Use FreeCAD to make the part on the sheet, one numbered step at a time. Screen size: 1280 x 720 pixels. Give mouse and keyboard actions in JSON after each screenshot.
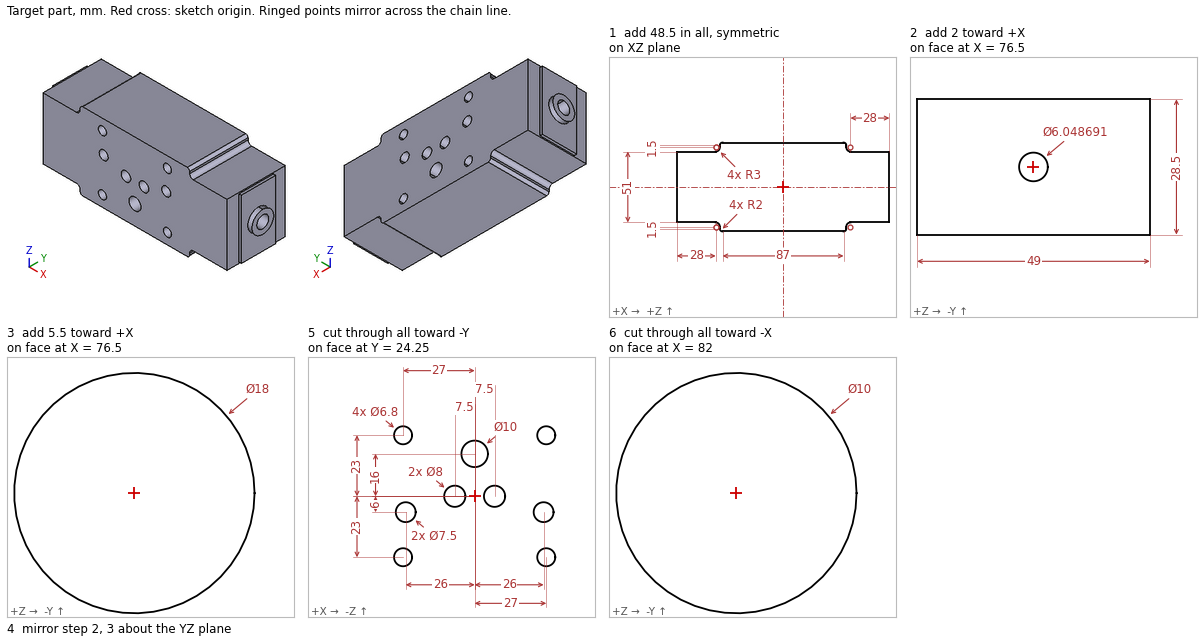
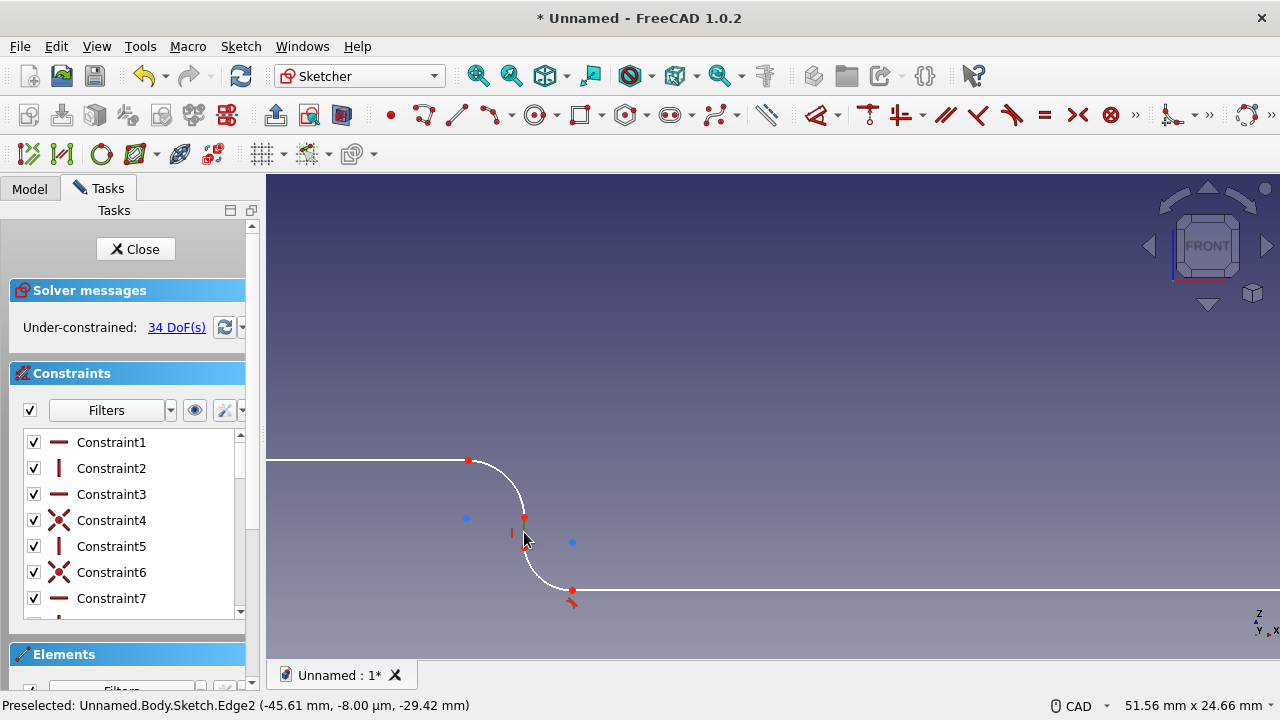
{"action": "left_click", "coordinate": [531, 567]}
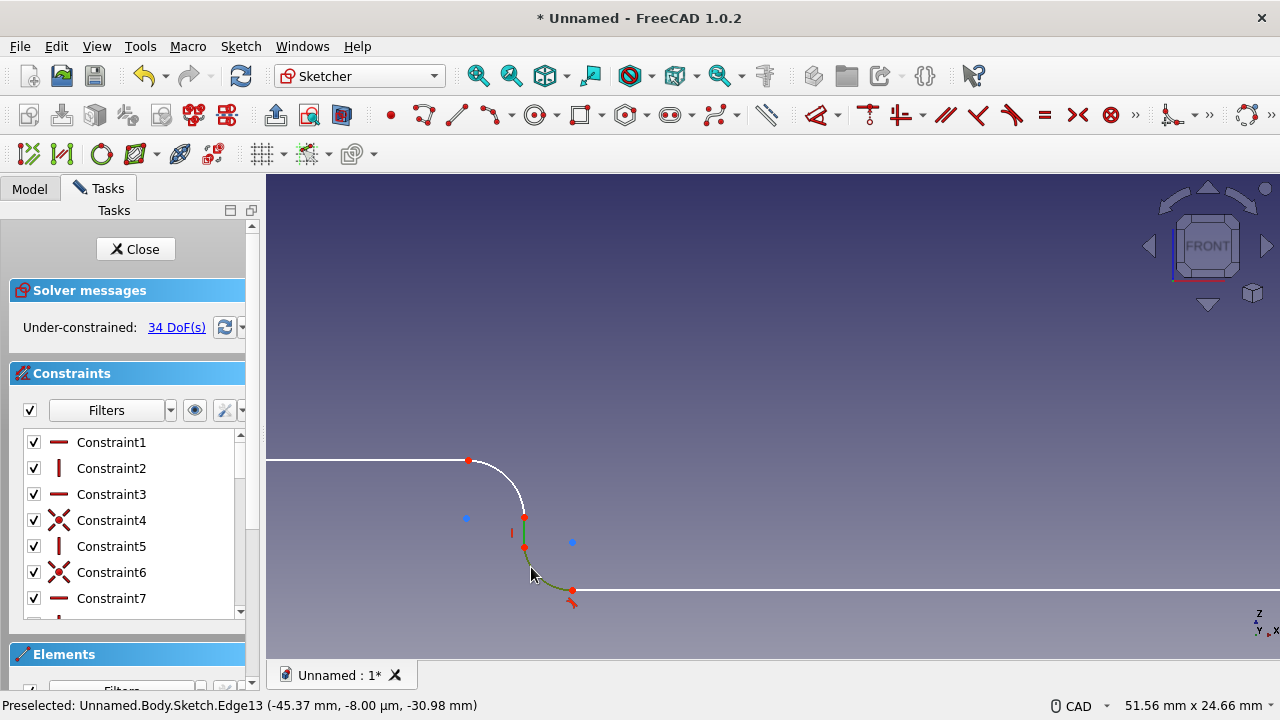
{"action": "left_click", "coordinate": [1012, 116]}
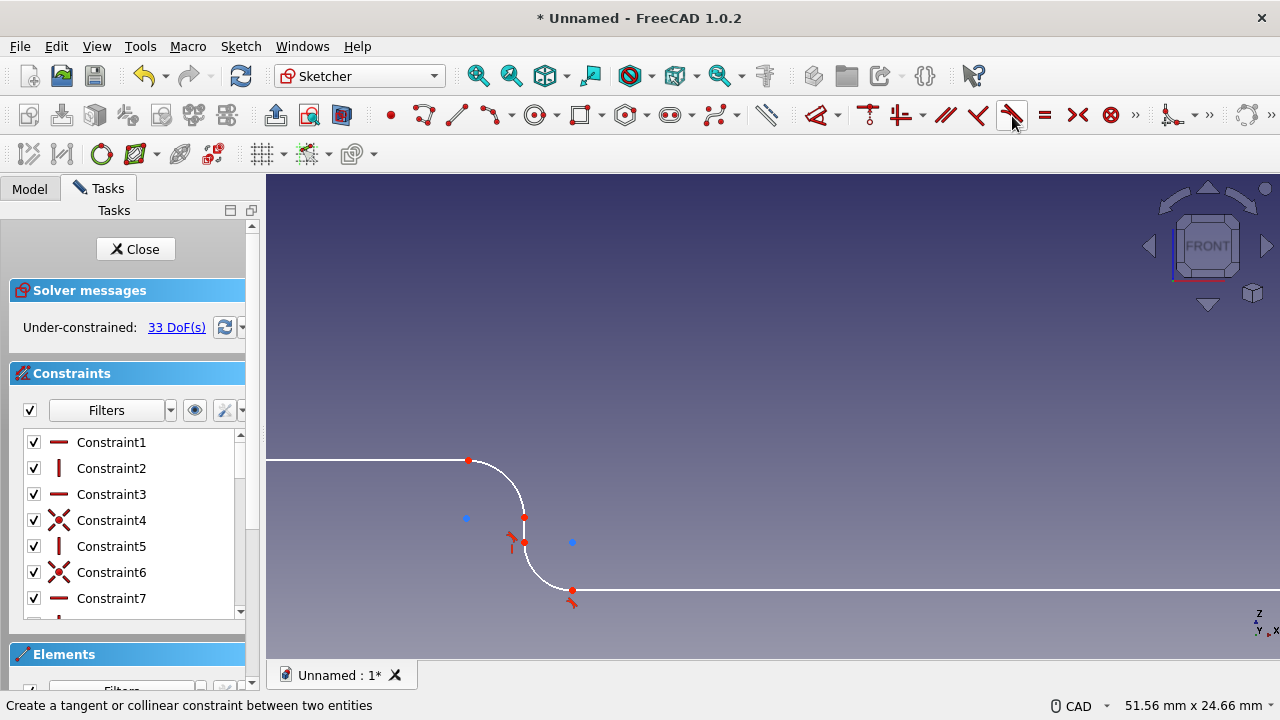
{"action": "scroll", "coordinate": [524, 532], "scroll_direction": "up", "scroll_amount": 2}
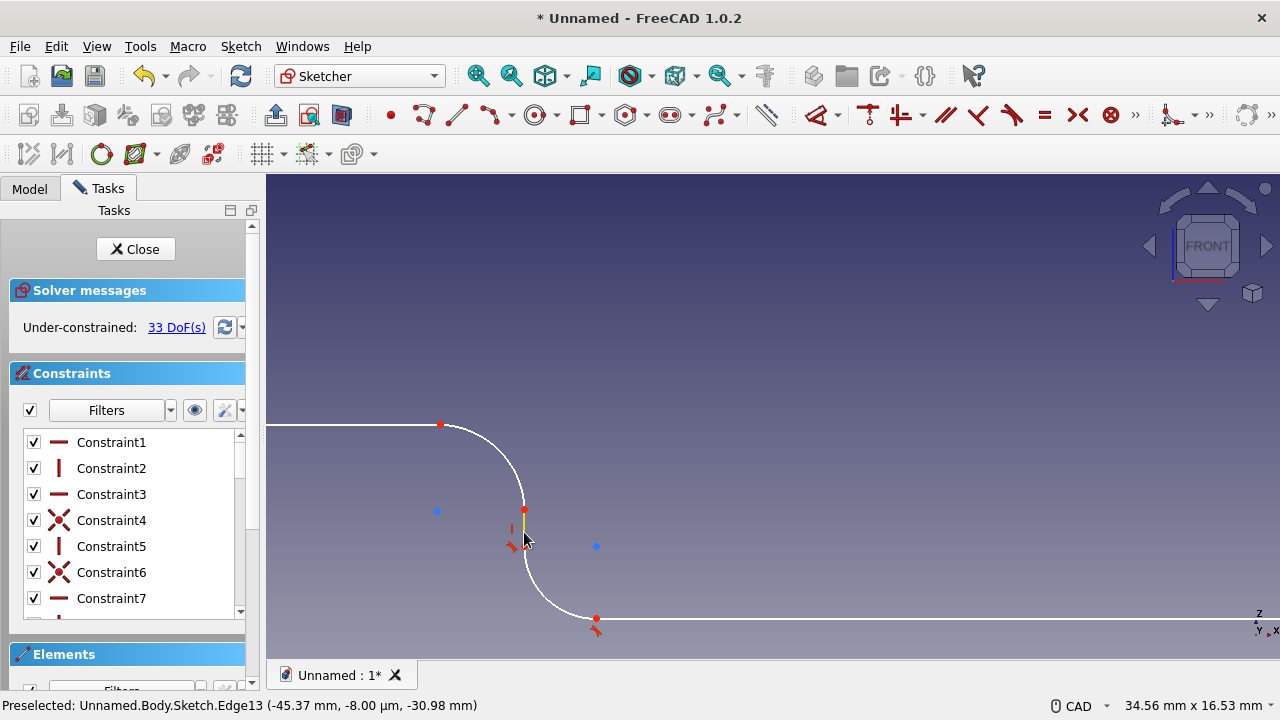
{"action": "left_click", "coordinate": [524, 532]}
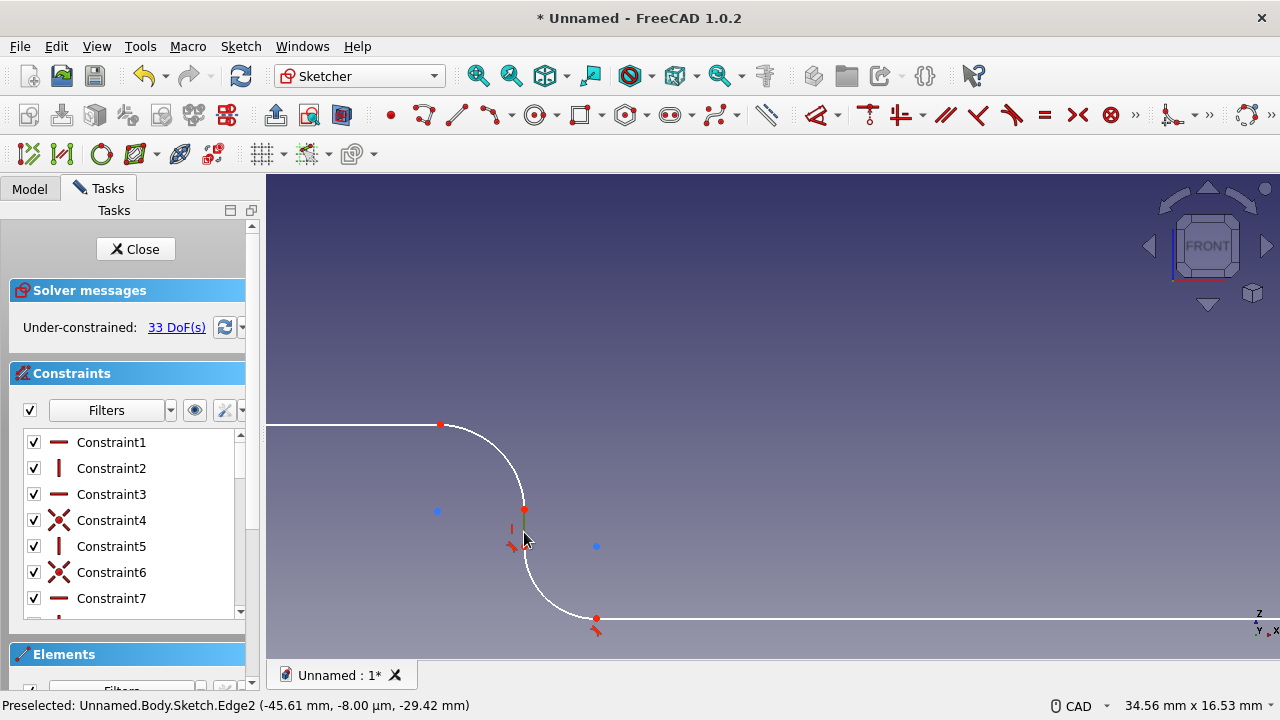
{"action": "left_click", "coordinate": [515, 472]}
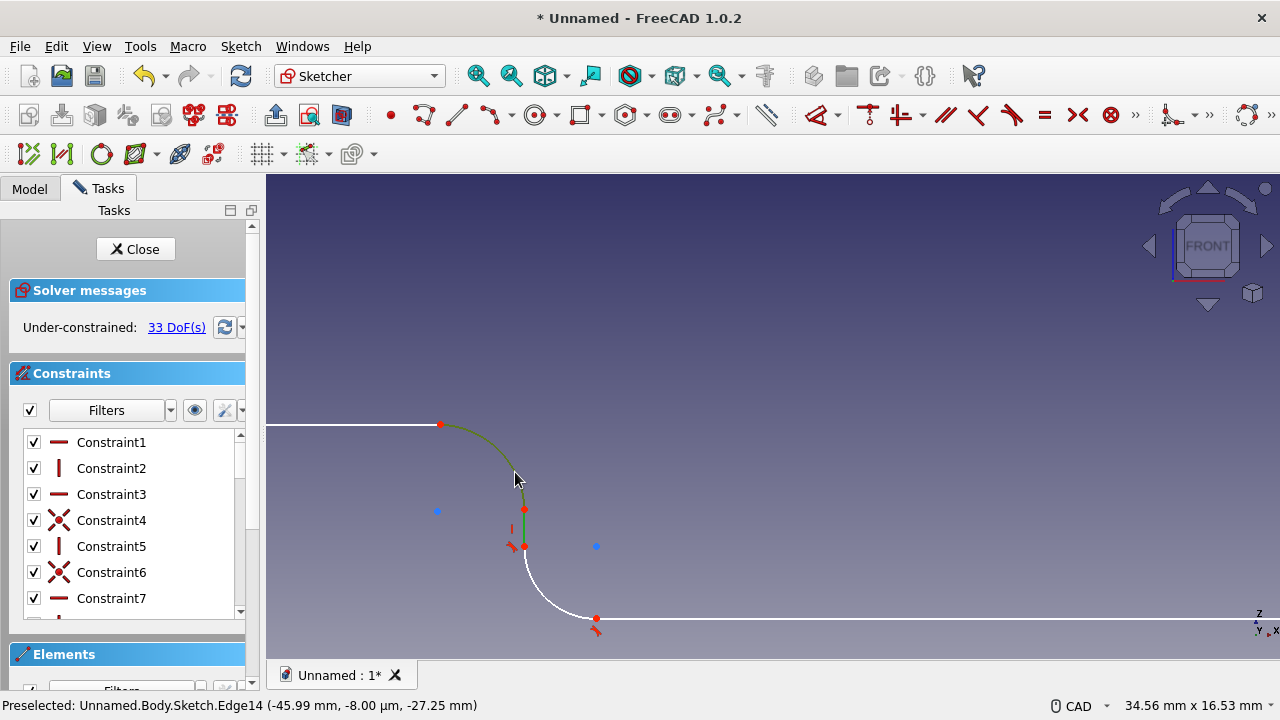
{"action": "left_click", "coordinate": [1012, 116]}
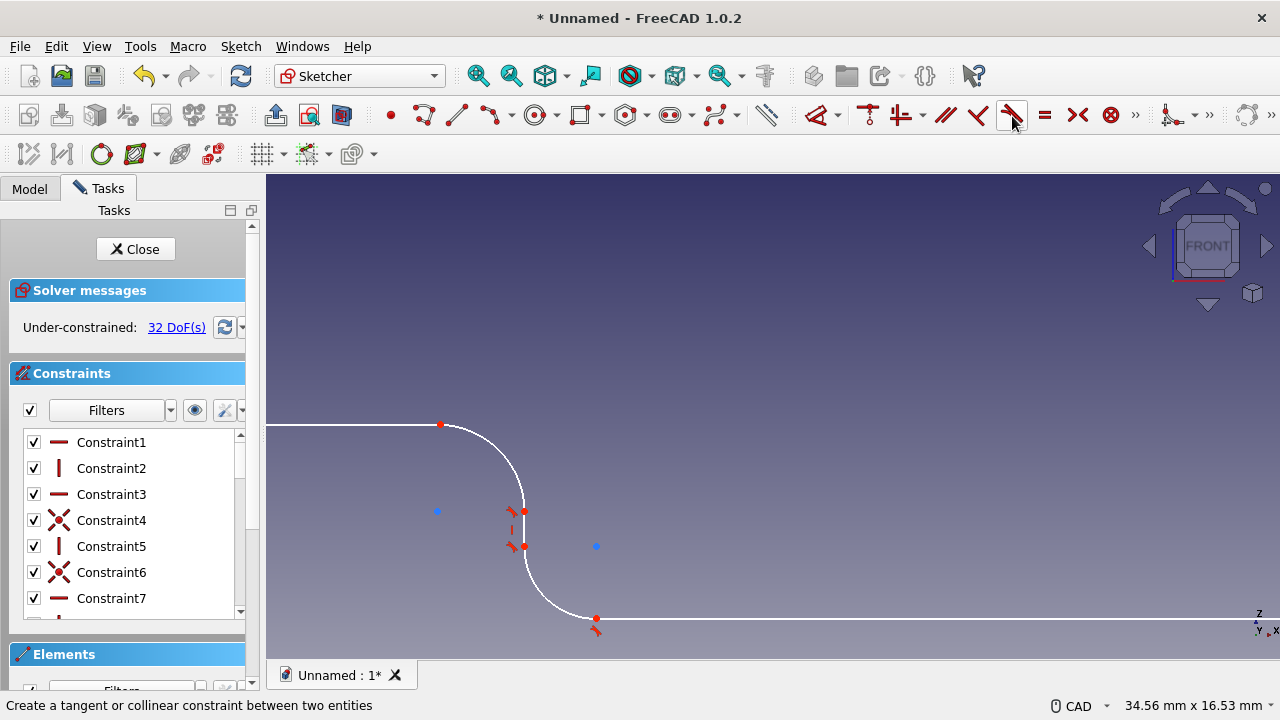
{"action": "scroll", "coordinate": [523, 533], "scroll_direction": "down", "scroll_amount": 10}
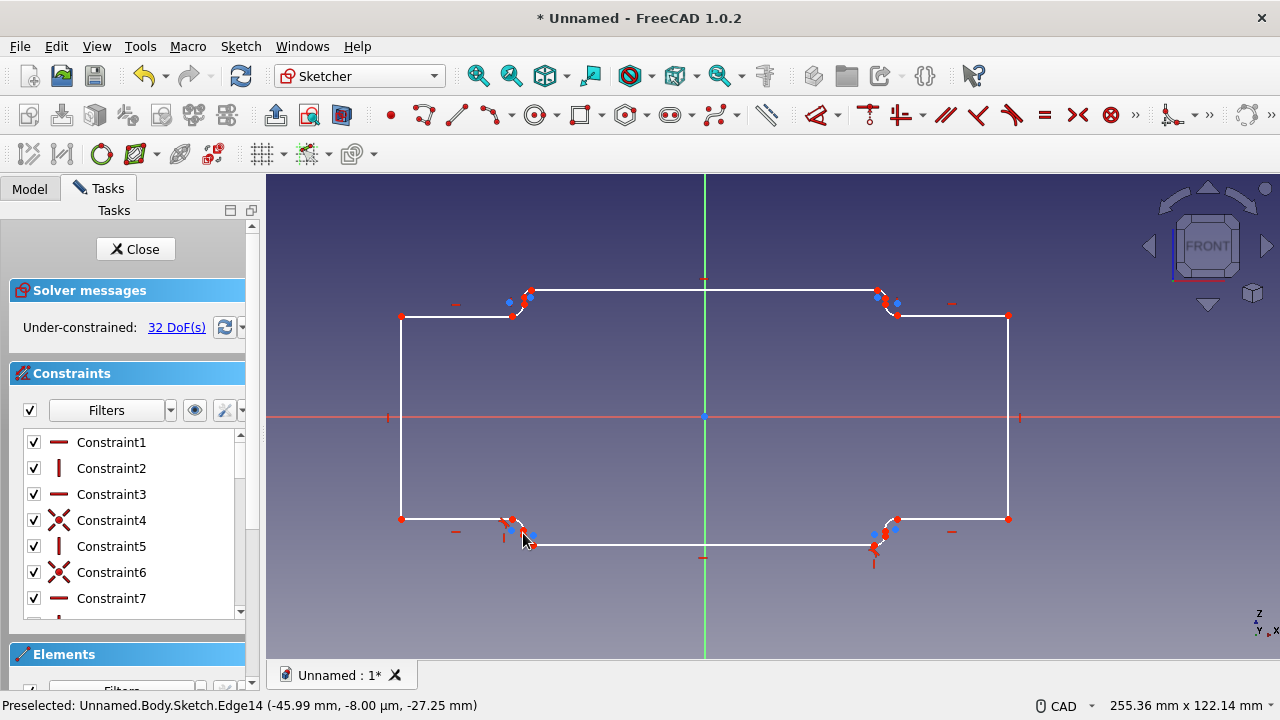
{"action": "left_click", "coordinate": [479, 519]}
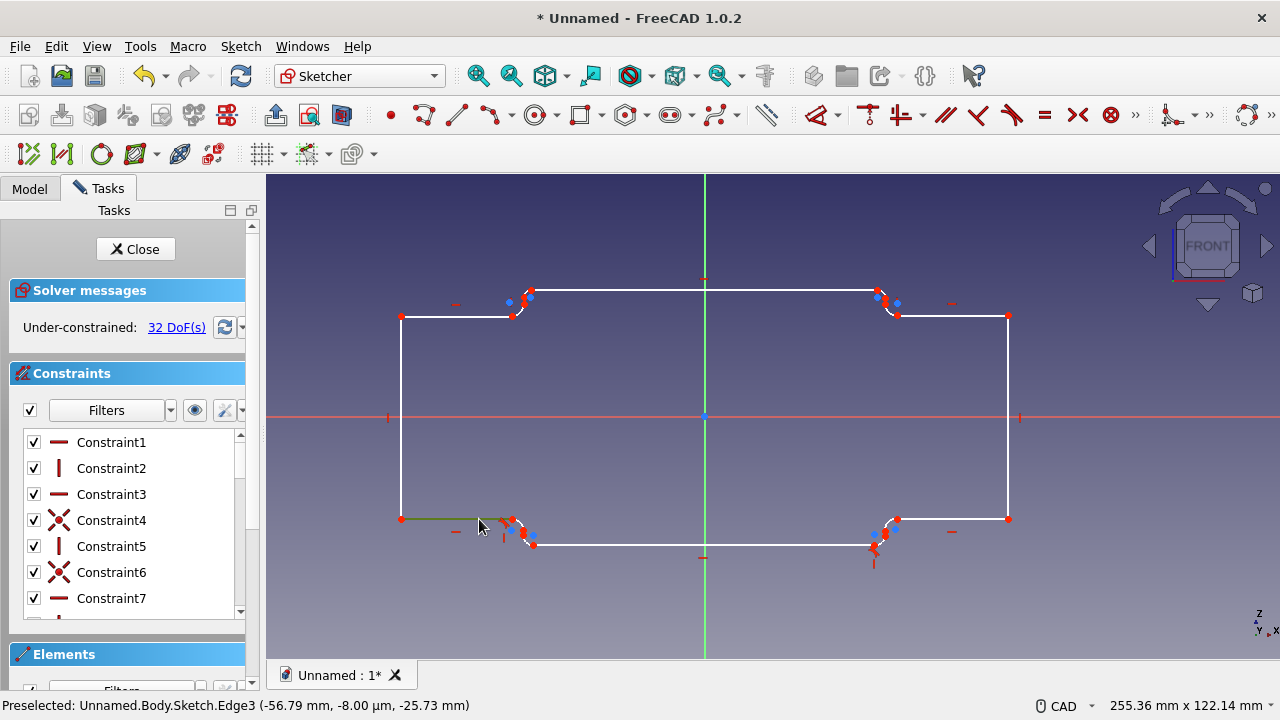
{"action": "scroll", "coordinate": [520, 523], "scroll_direction": "up", "scroll_amount": 3}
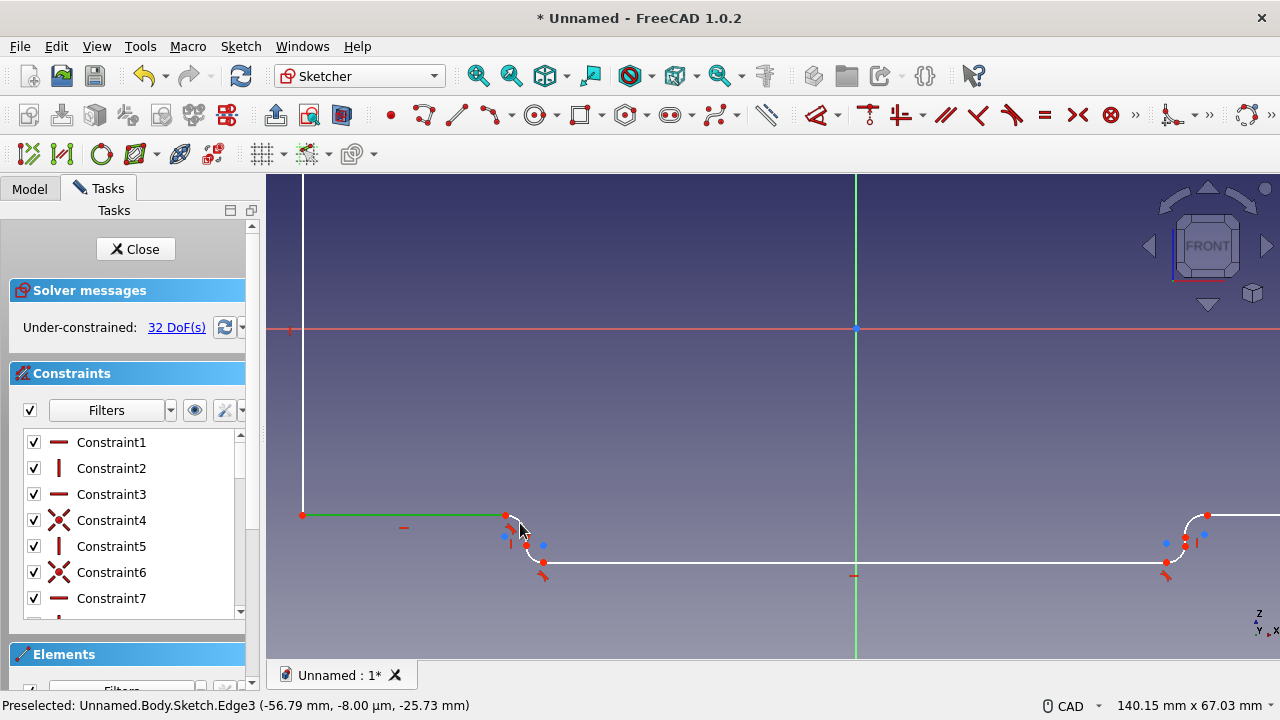
{"action": "left_click", "coordinate": [520, 522]}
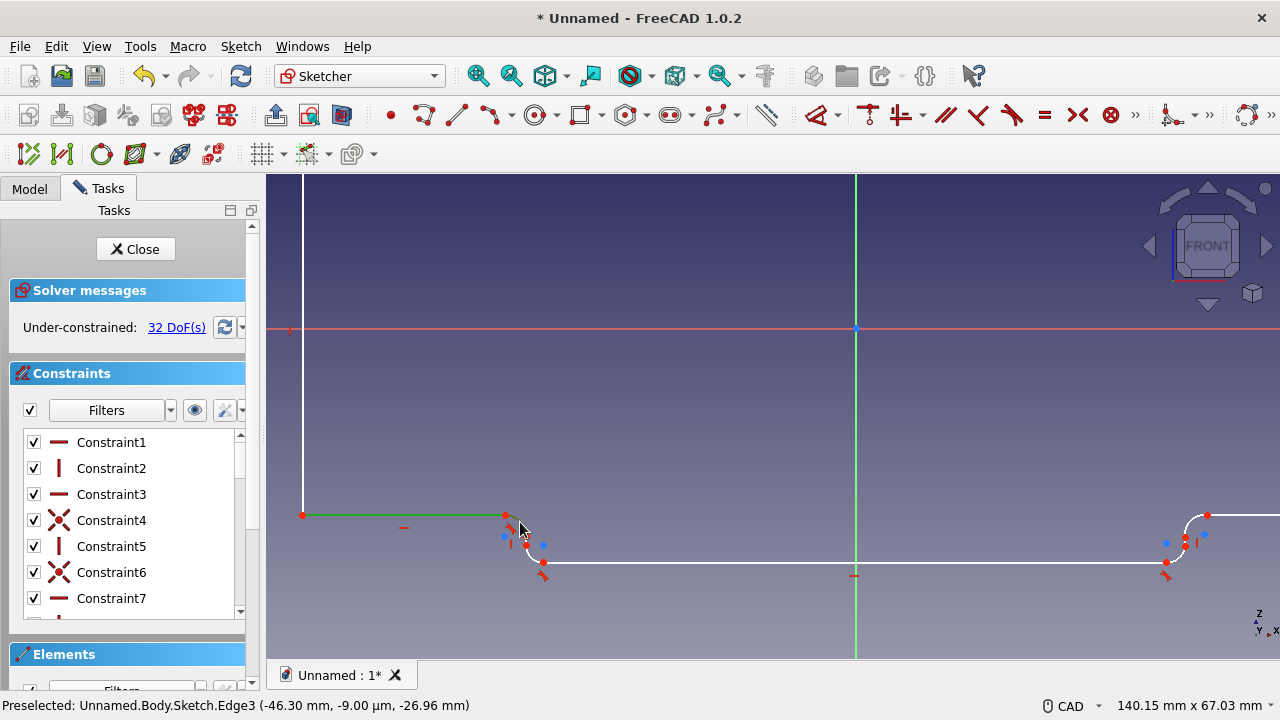
{"action": "left_click", "coordinate": [1012, 116]}